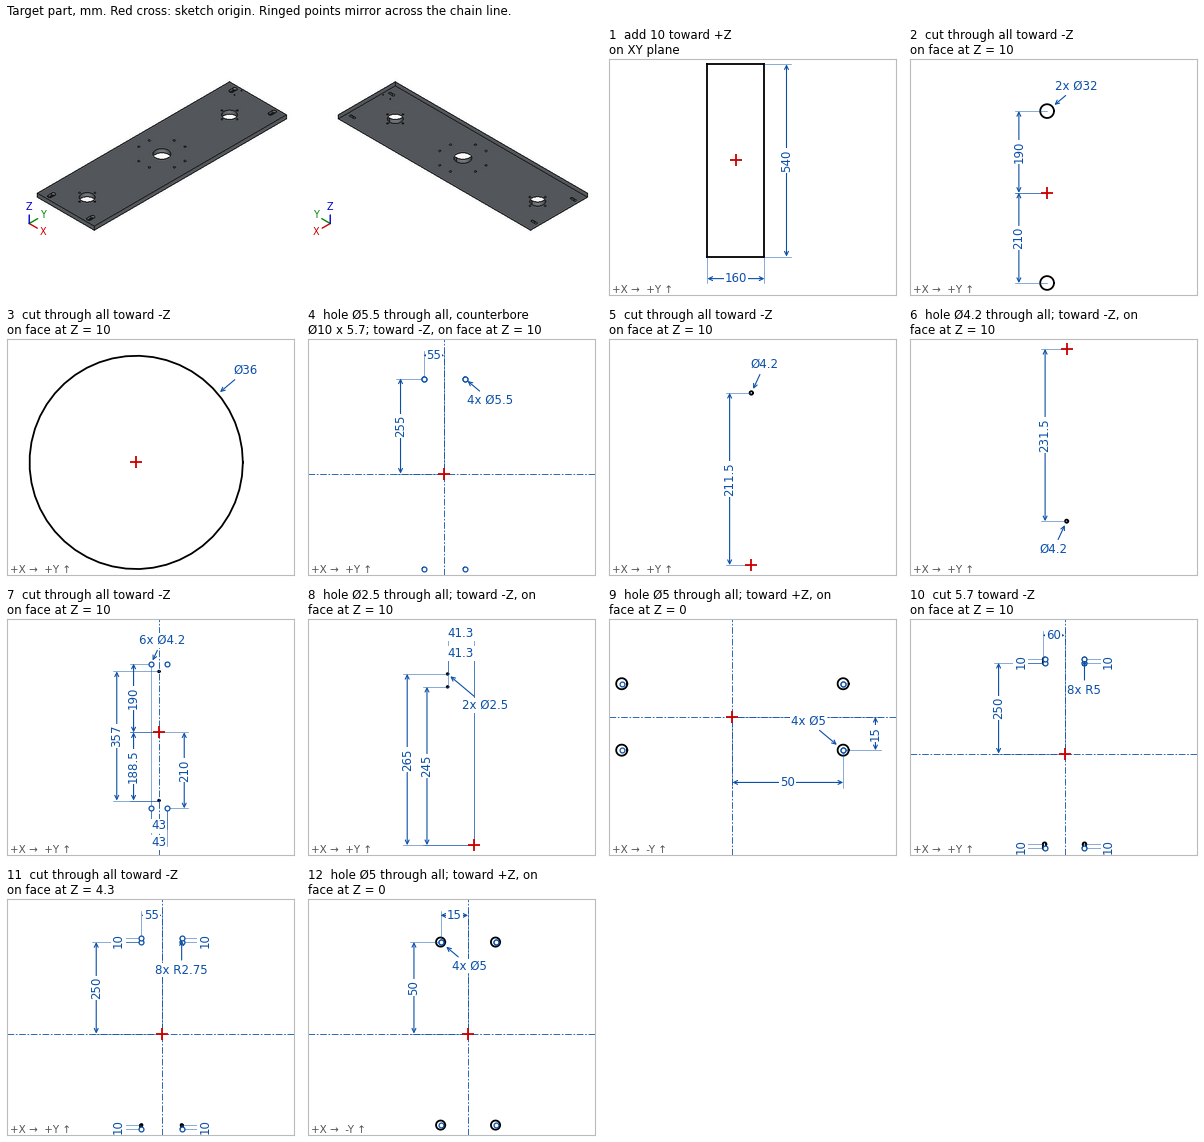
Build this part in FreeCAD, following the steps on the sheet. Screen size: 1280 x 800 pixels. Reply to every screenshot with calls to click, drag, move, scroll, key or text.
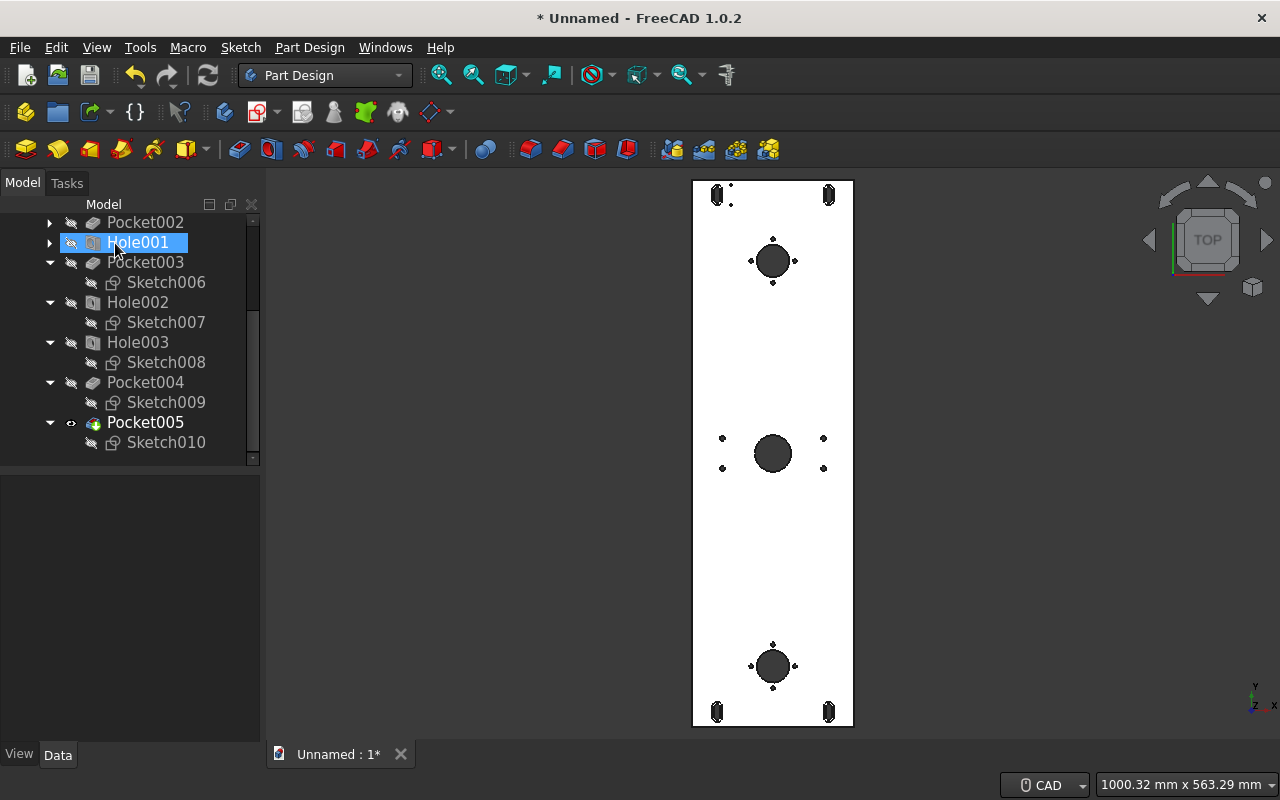
key(5)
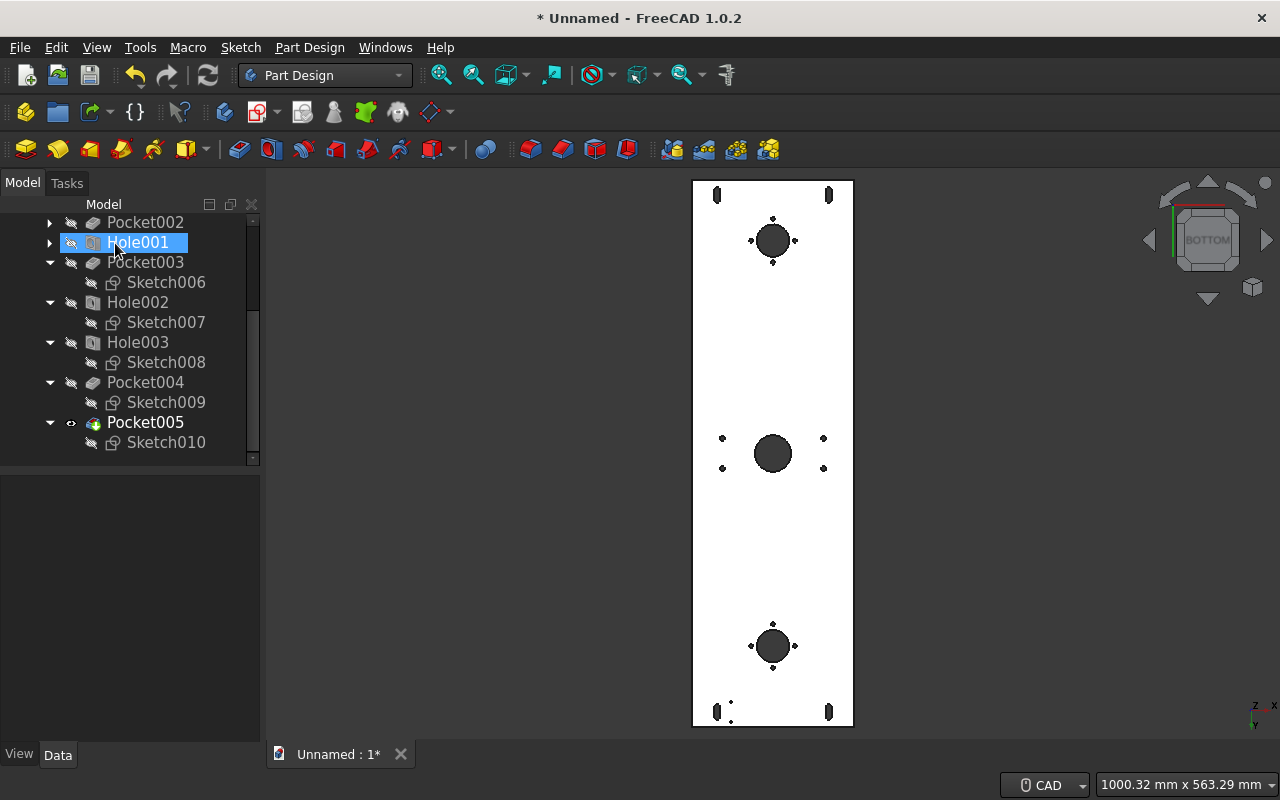
click(773, 531)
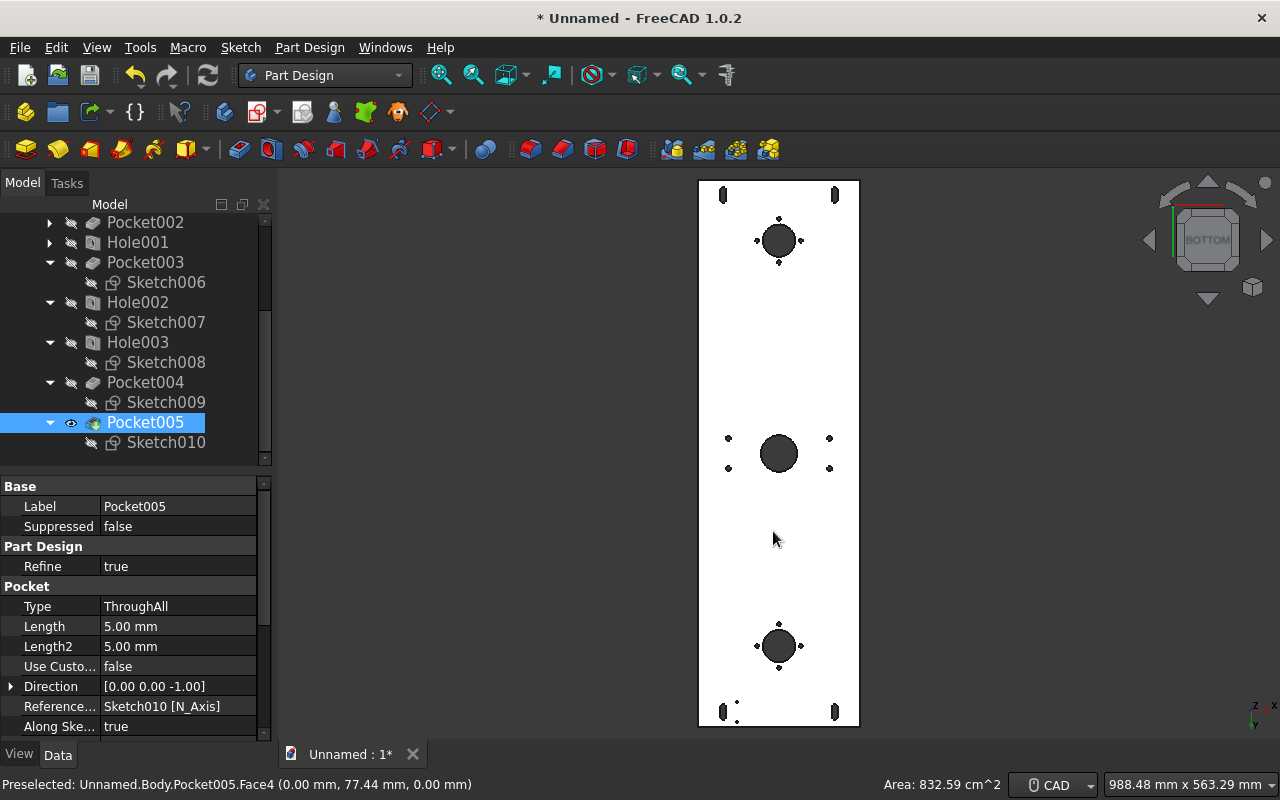
click(258, 112)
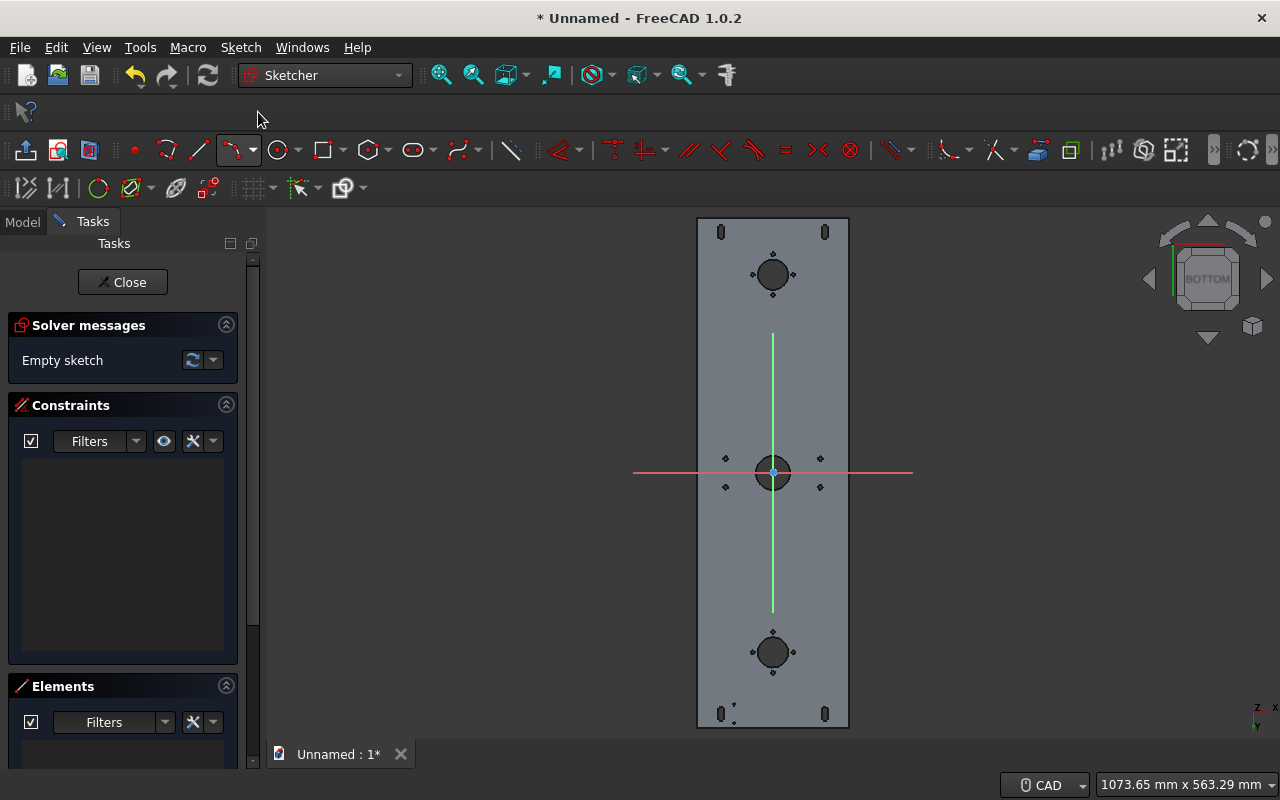
scroll(803, 473, up, 6)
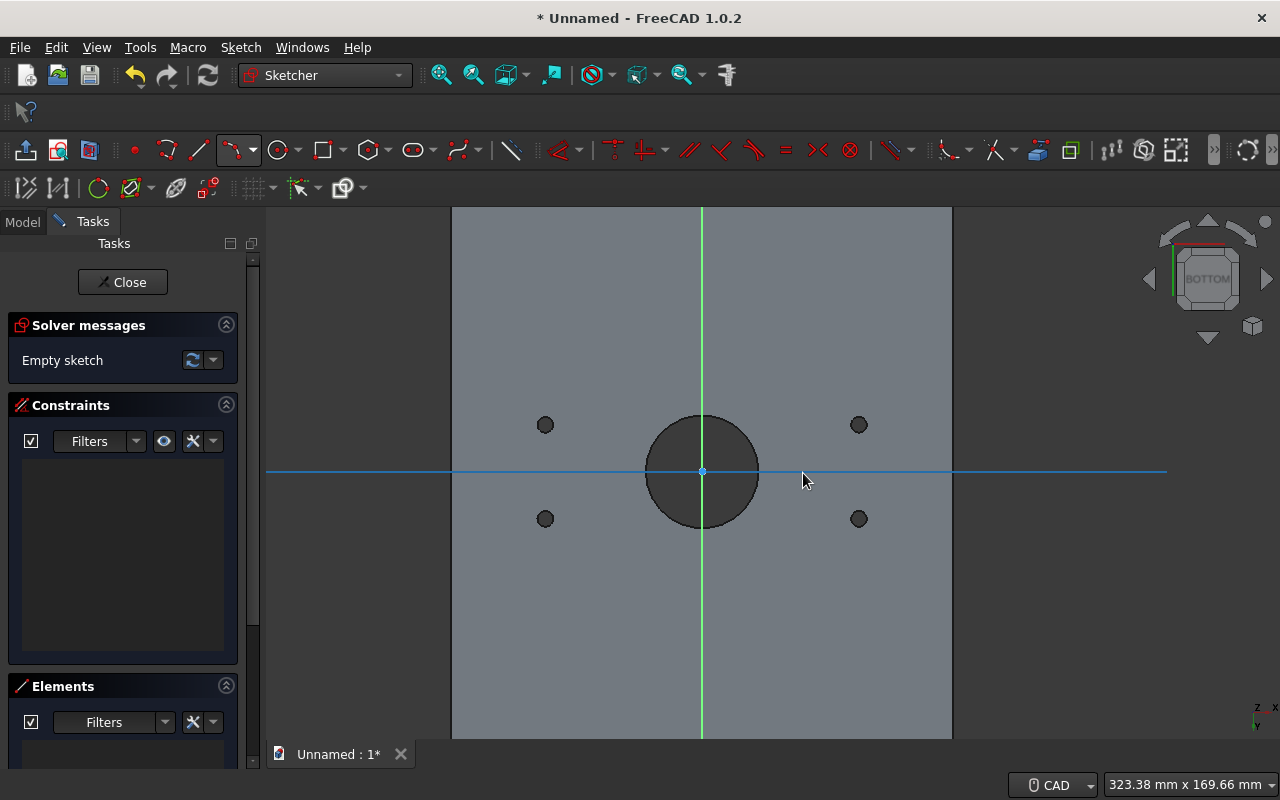
key(g)
key(c)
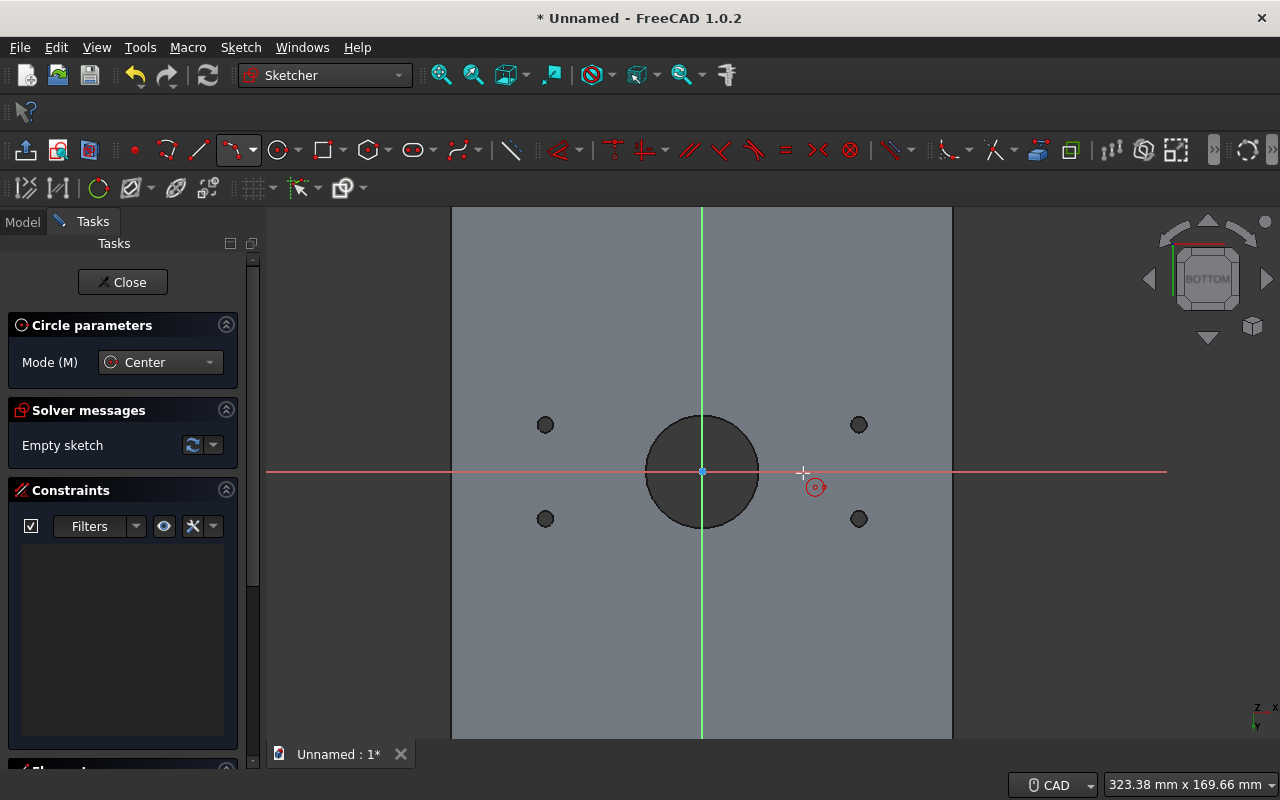
scroll(655, 315, up, 6)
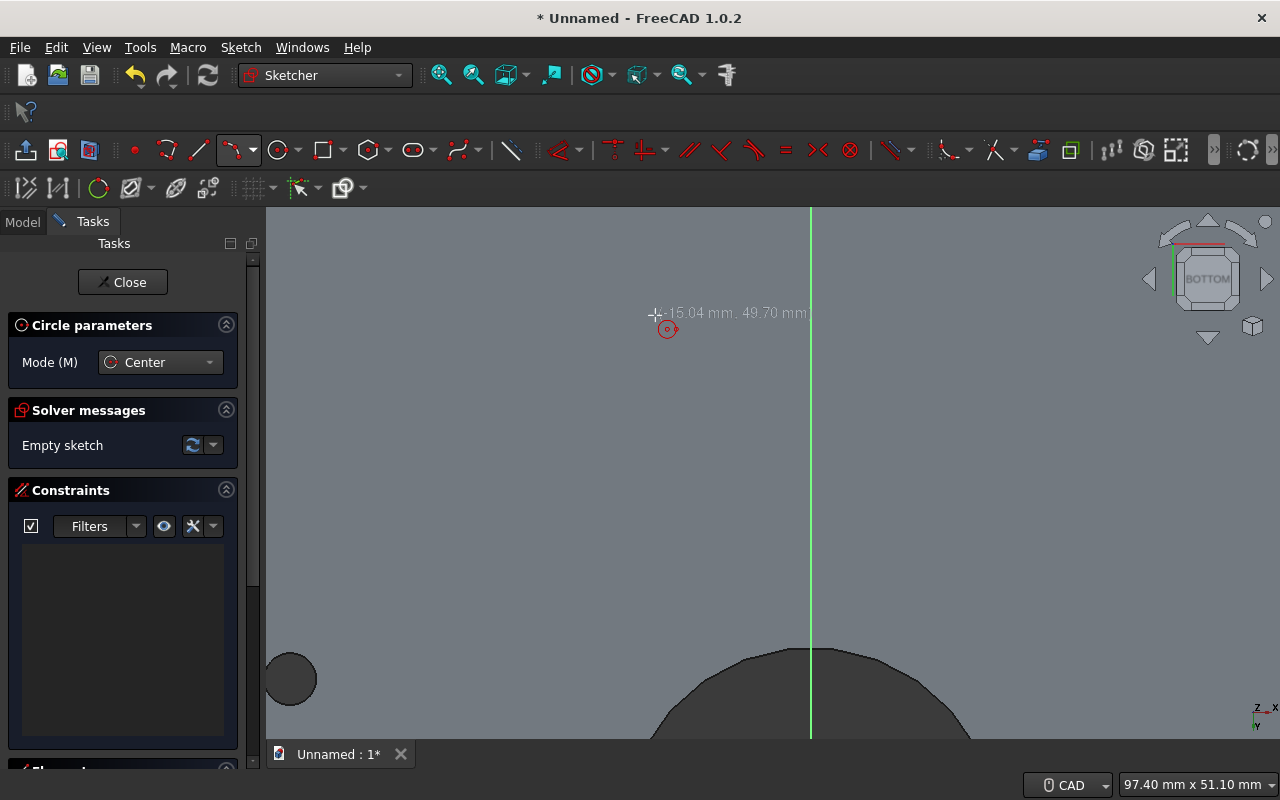
click(655, 315)
move(673, 296)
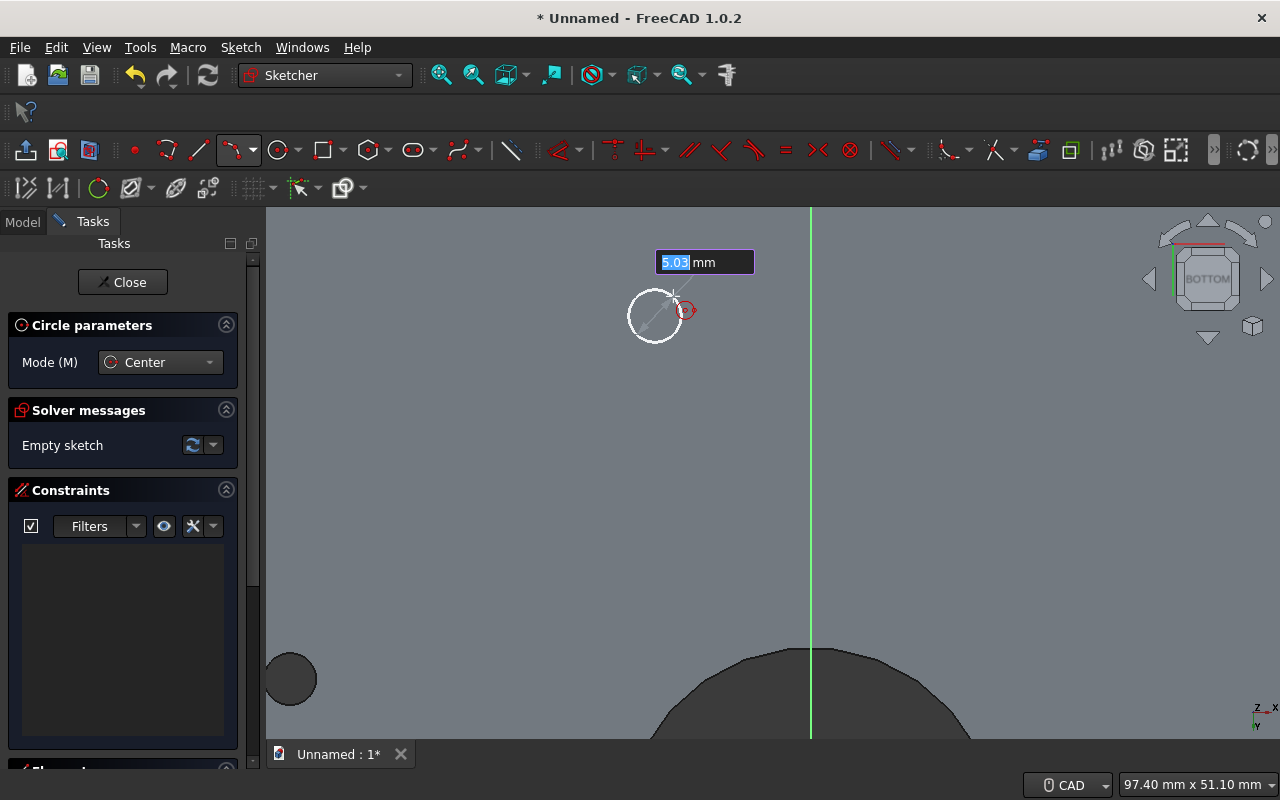
text(5)
key(Return)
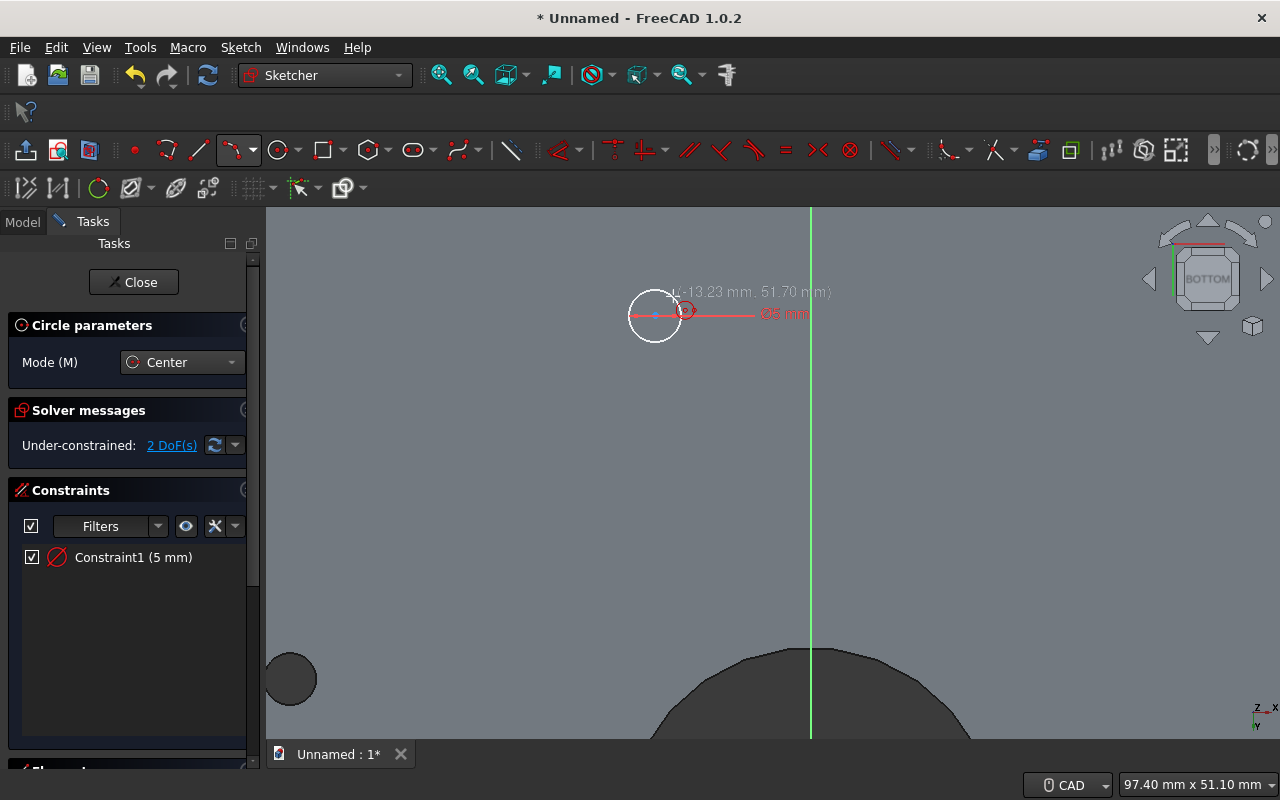
click(967, 315)
move(985, 296)